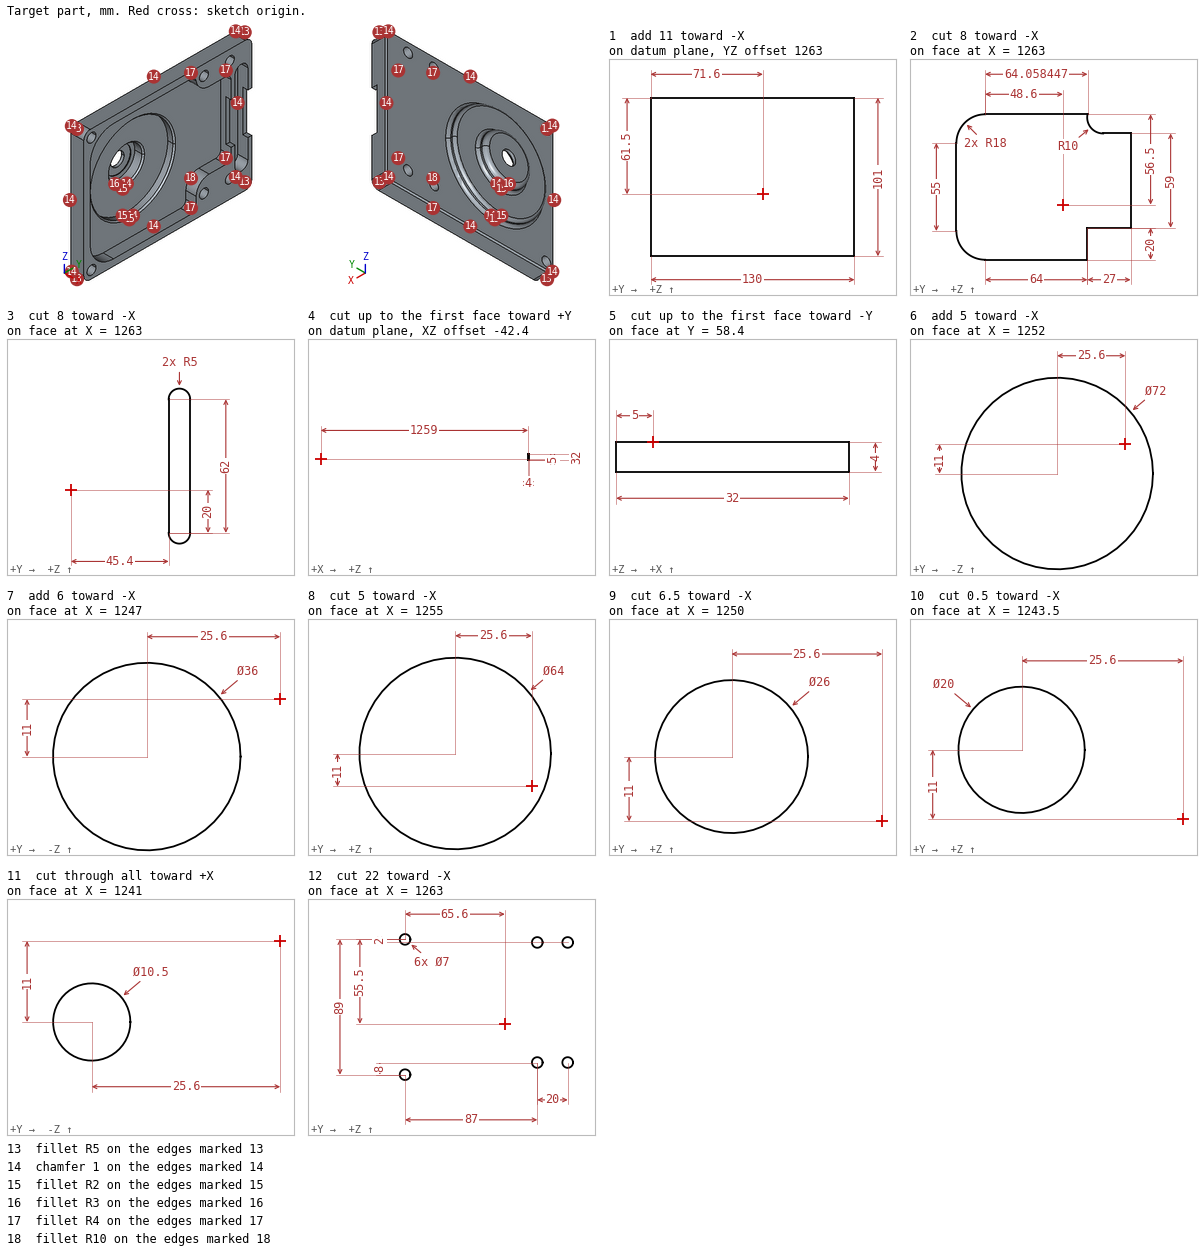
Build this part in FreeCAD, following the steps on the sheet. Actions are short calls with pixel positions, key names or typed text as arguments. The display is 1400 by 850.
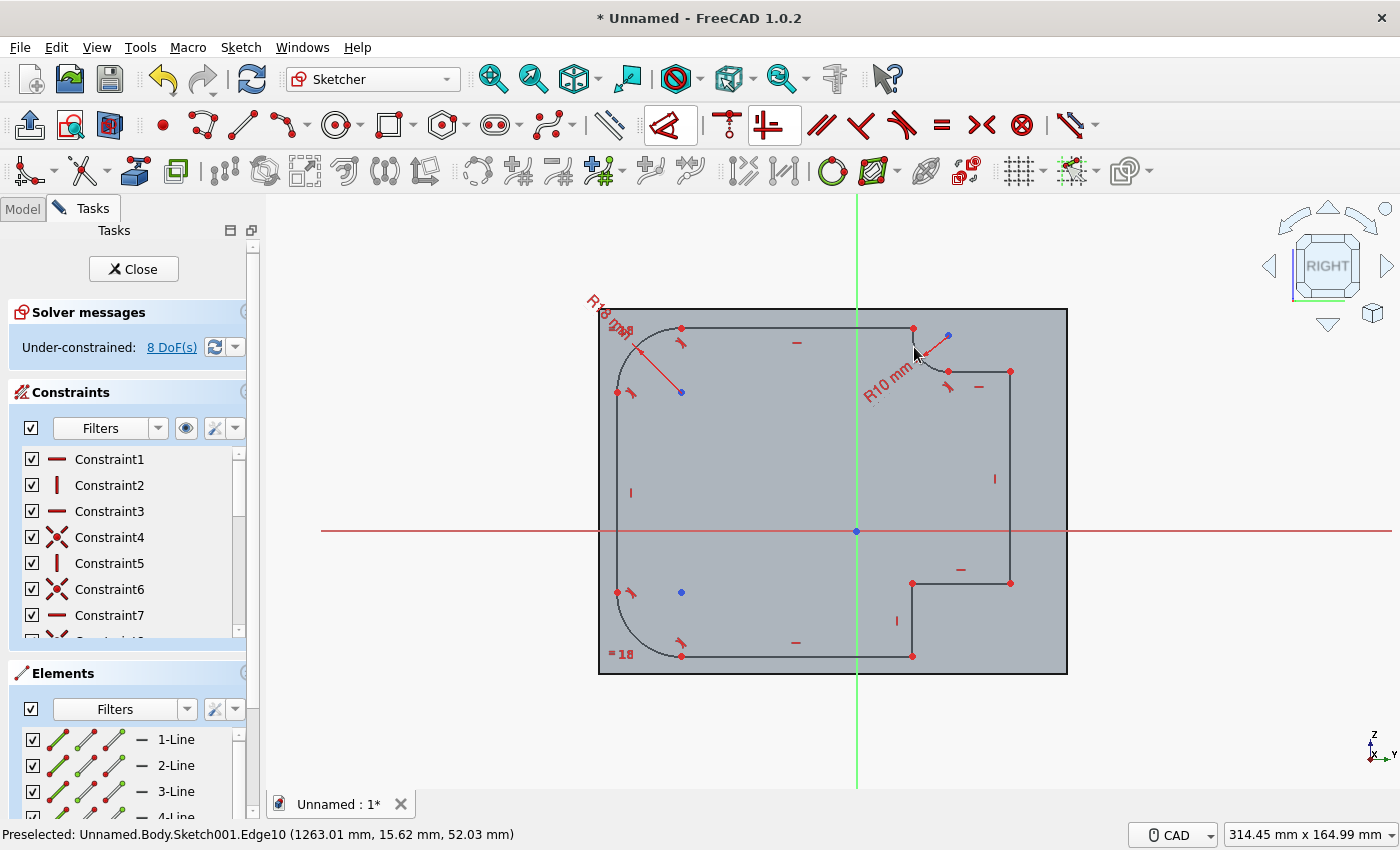
click(617, 453)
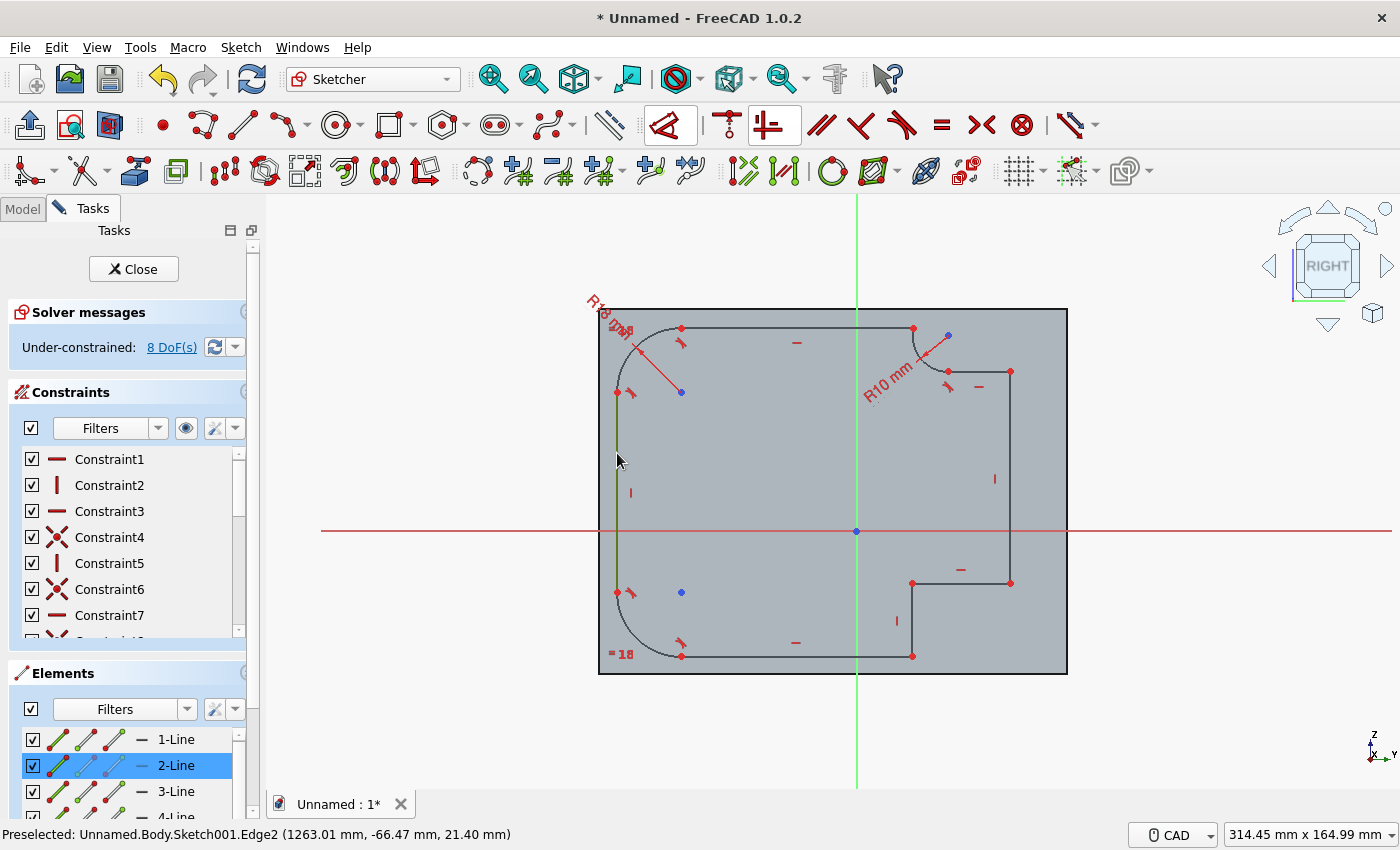
key(i)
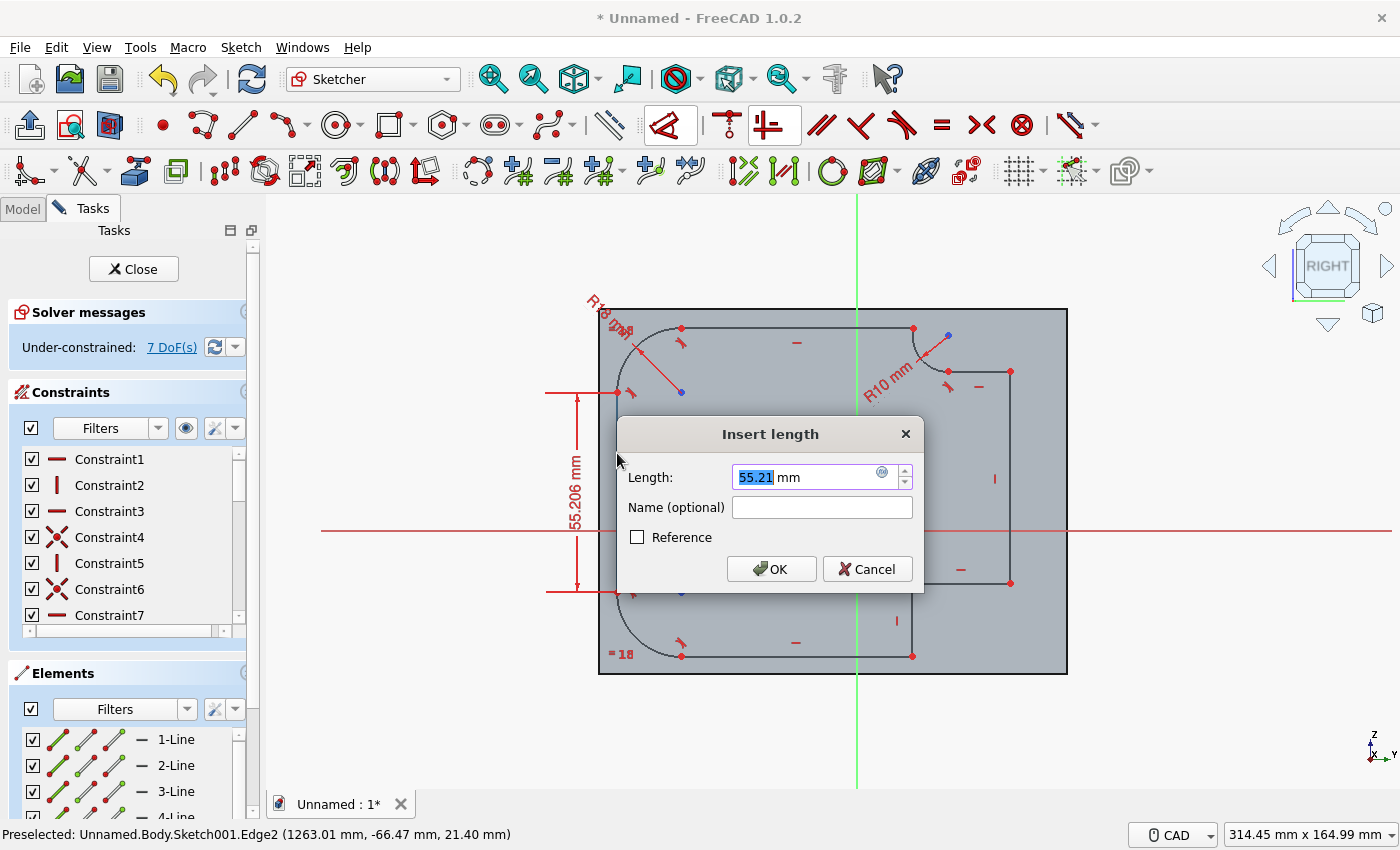
text(55)
key(Return)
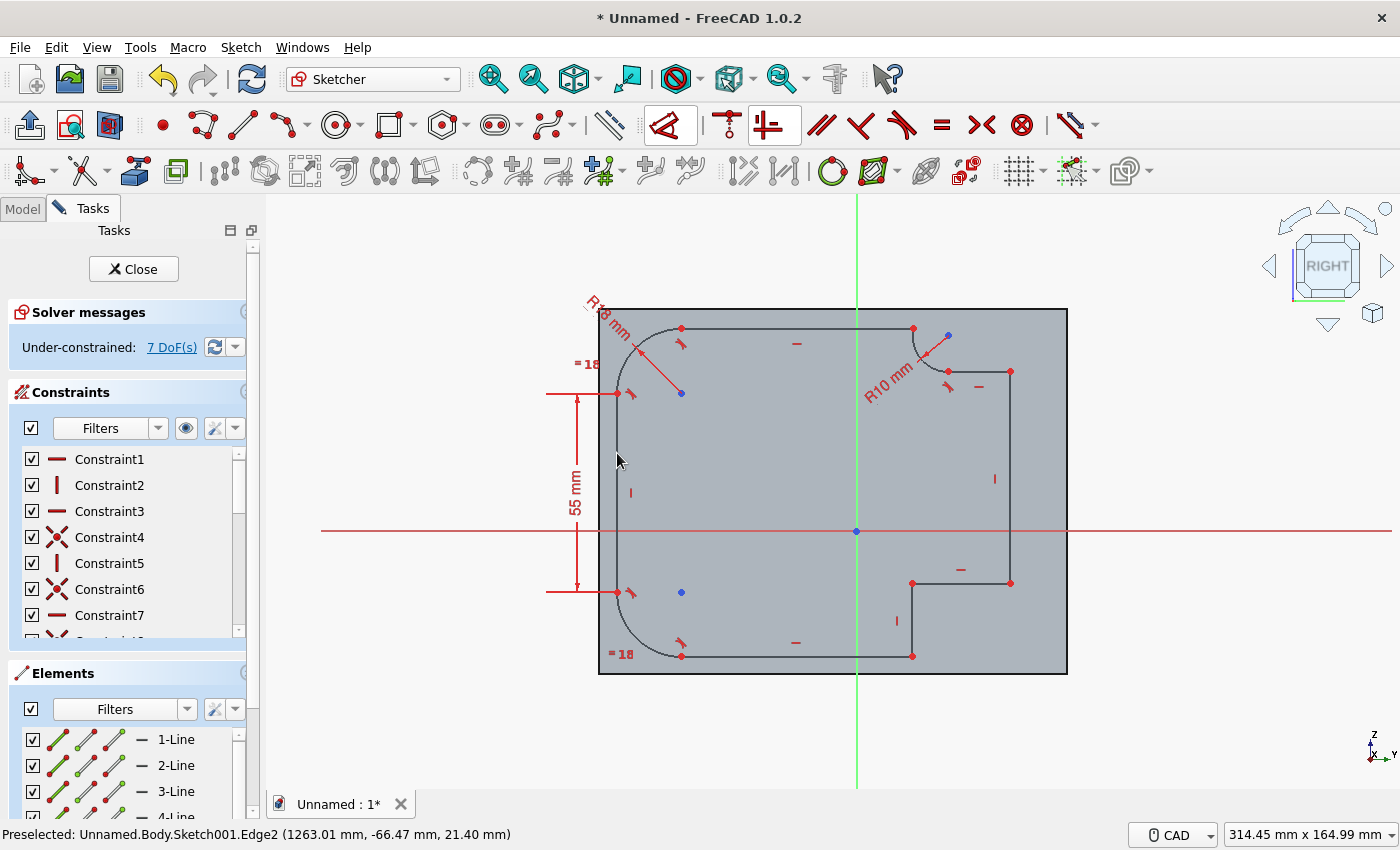
click(751, 657)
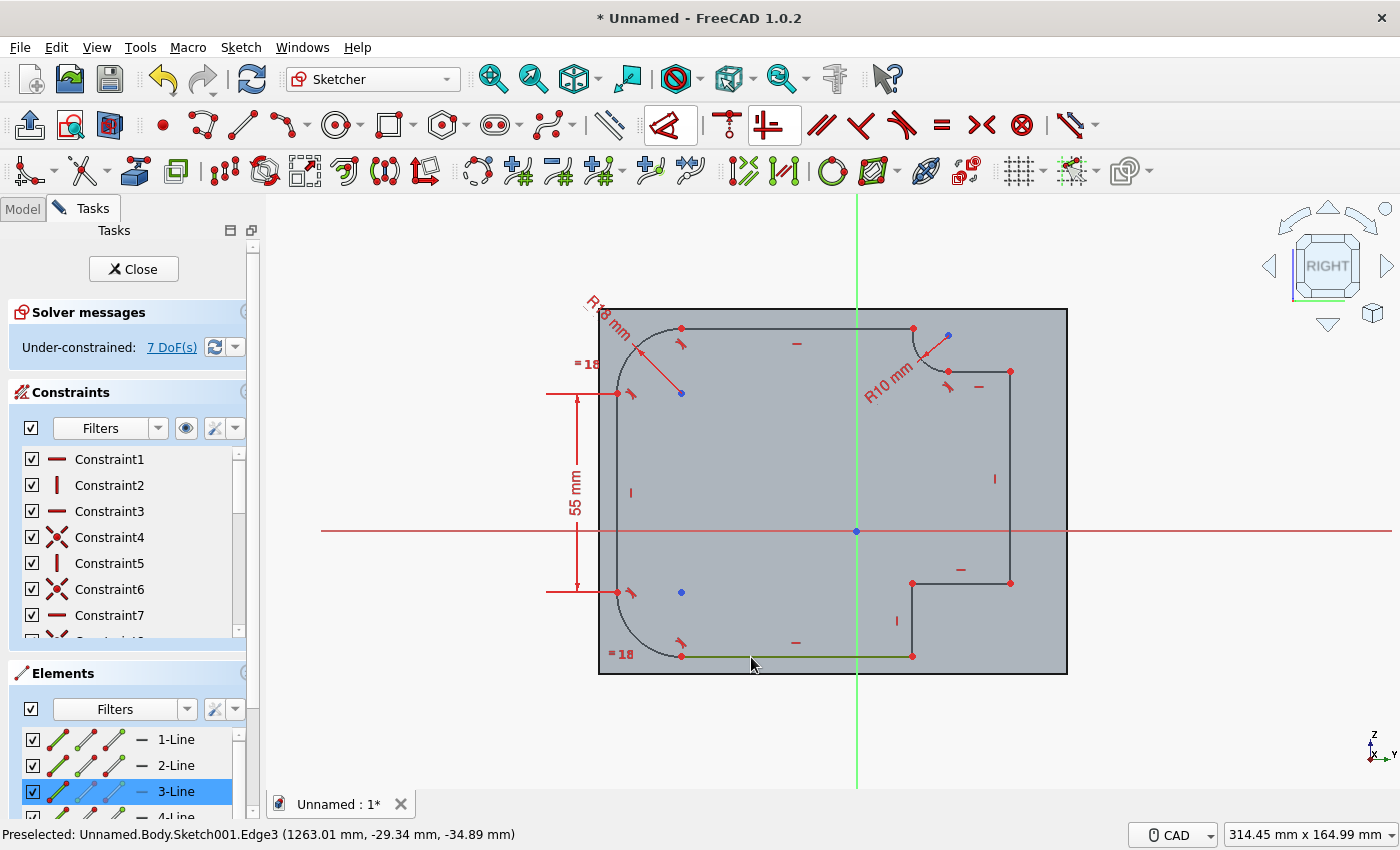
click(692, 126)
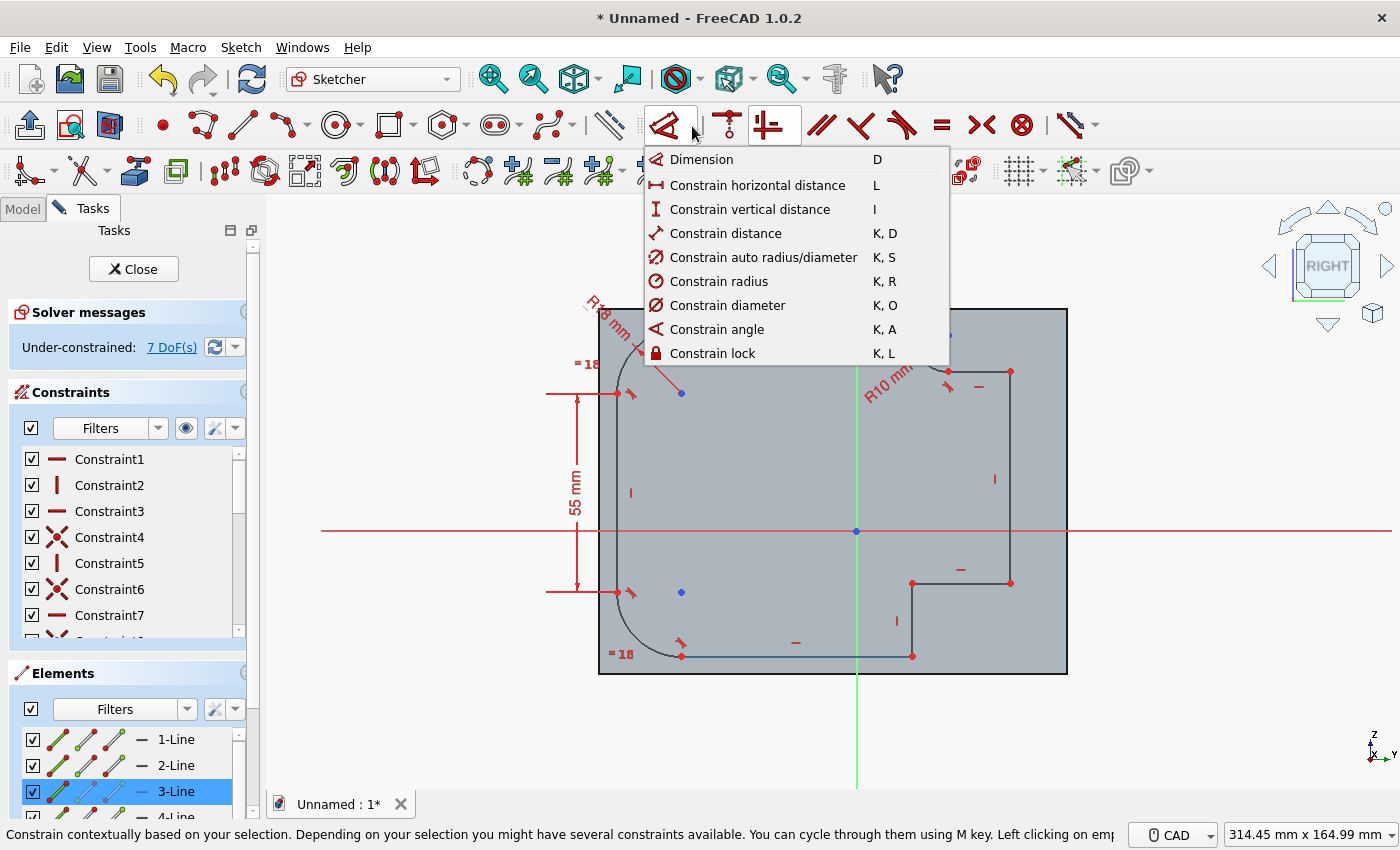
click(797, 185)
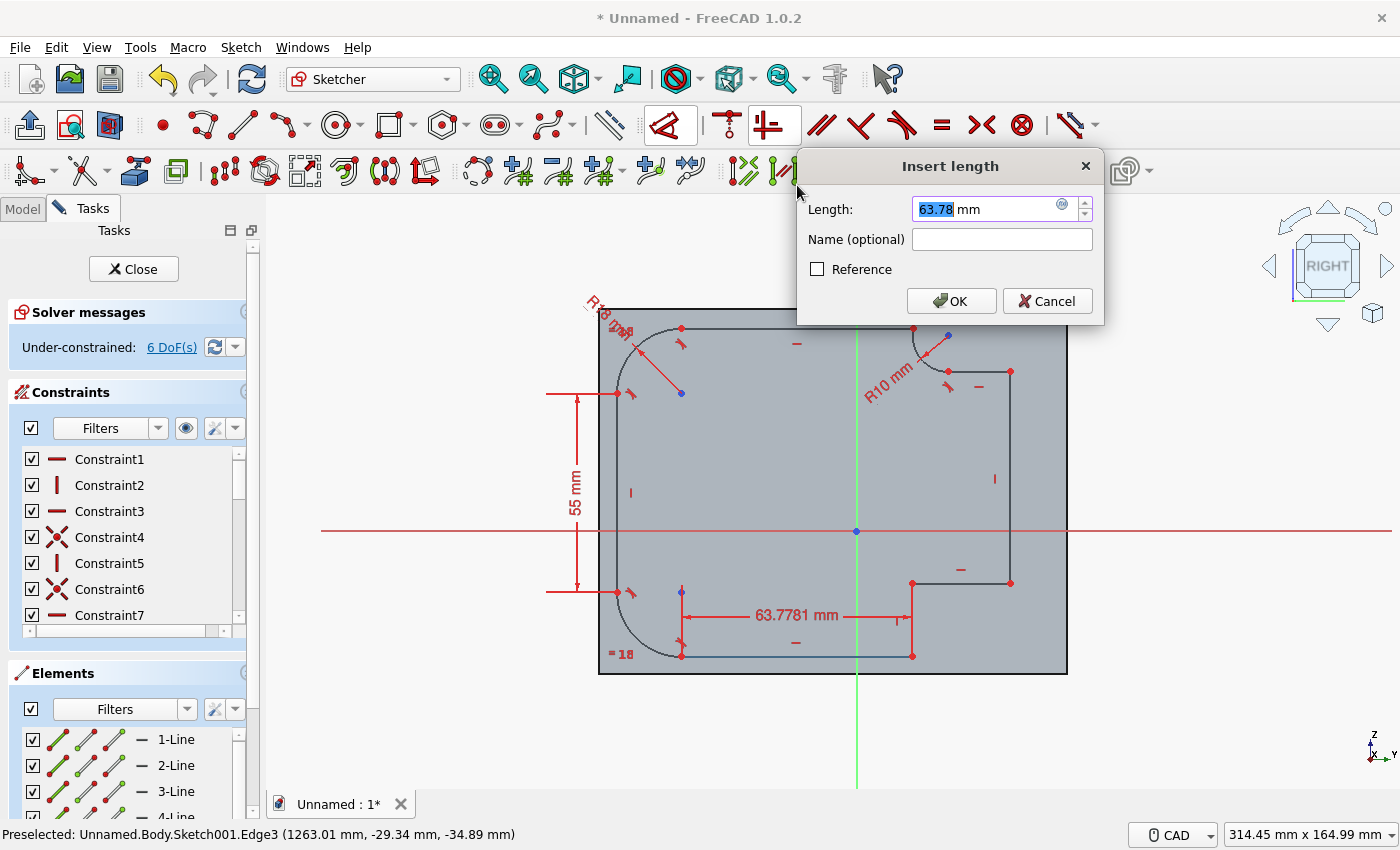
text(64)
key(Return)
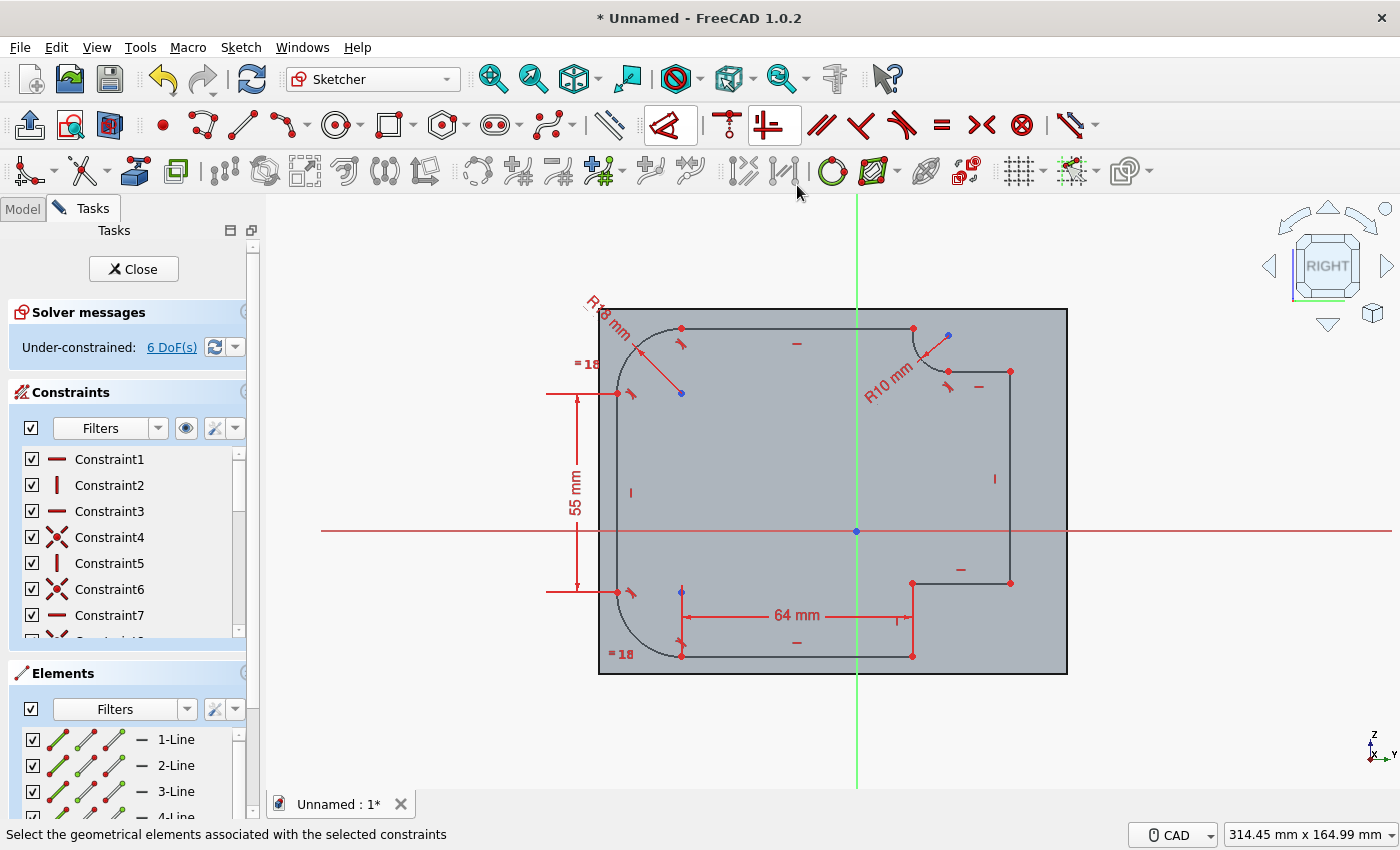
click(913, 635)